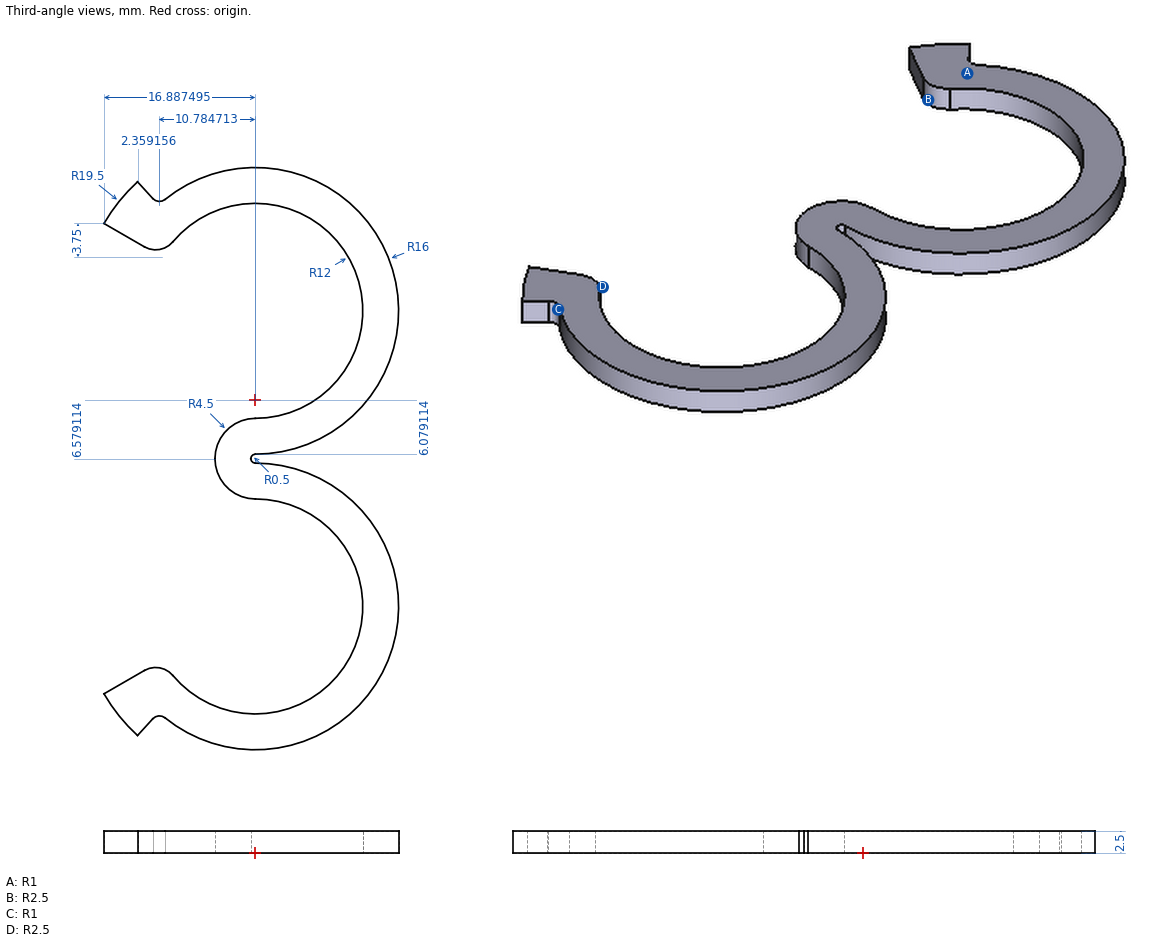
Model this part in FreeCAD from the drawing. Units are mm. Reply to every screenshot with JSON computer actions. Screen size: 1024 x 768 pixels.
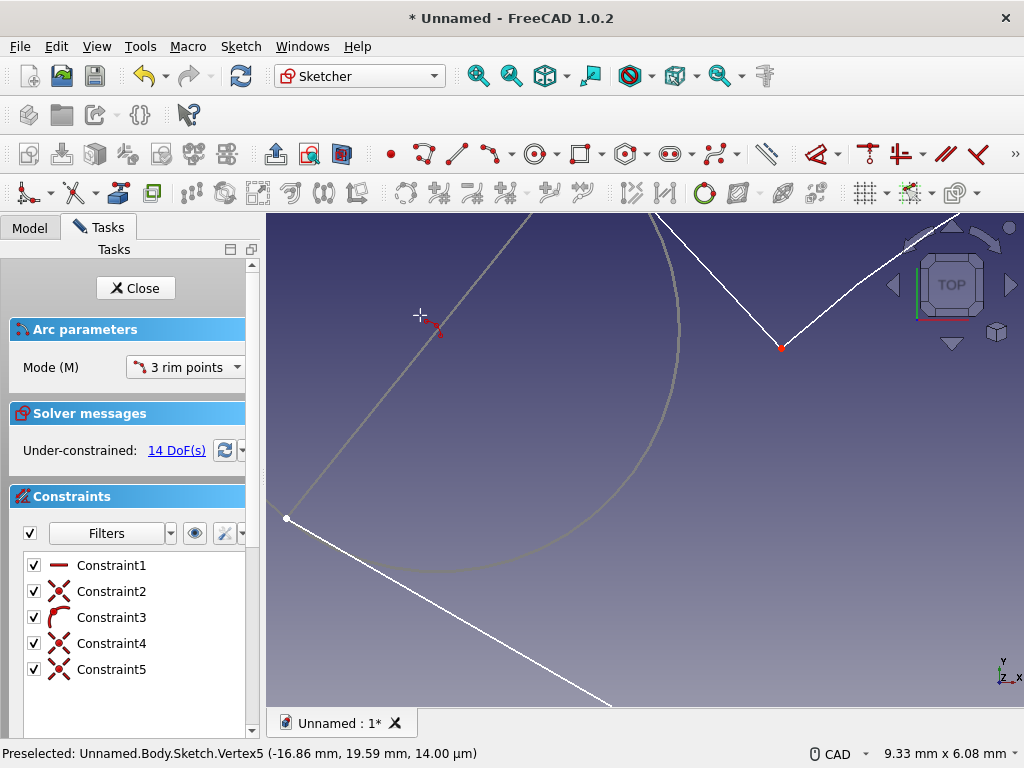
{"action": "left_click", "coordinate": [422, 311]}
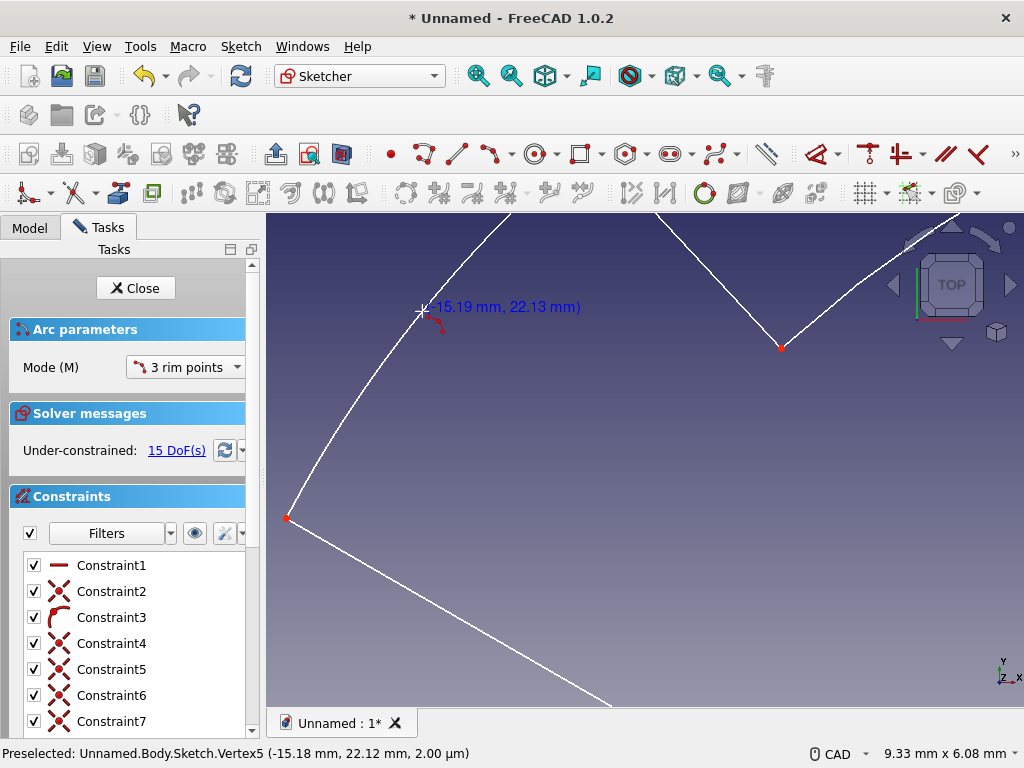
{"action": "scroll", "coordinate": [420, 315], "scroll_direction": "down", "scroll_amount": 10}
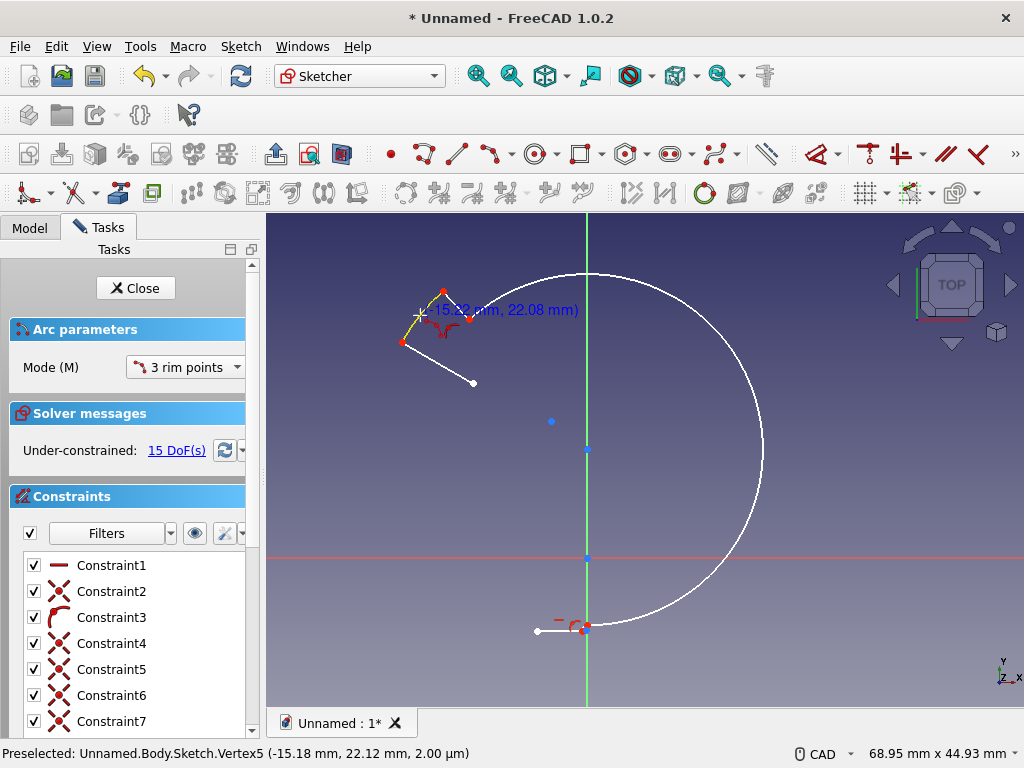
{"action": "left_click", "coordinate": [473, 384]}
{"action": "left_click", "coordinate": [587, 581]}
{"action": "left_click", "coordinate": [702, 383]}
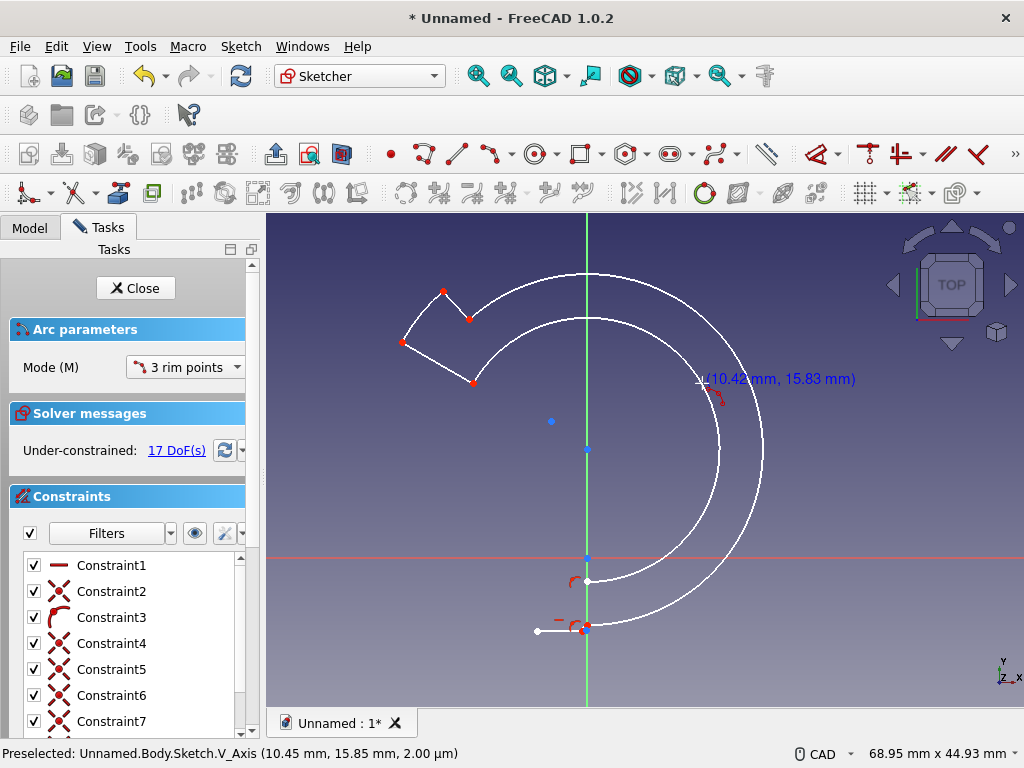
{"action": "left_click", "coordinate": [587, 582]}
{"action": "left_click", "coordinate": [538, 631]}
{"action": "left_click", "coordinate": [552, 595]}
{"action": "key", "text": "Escape"}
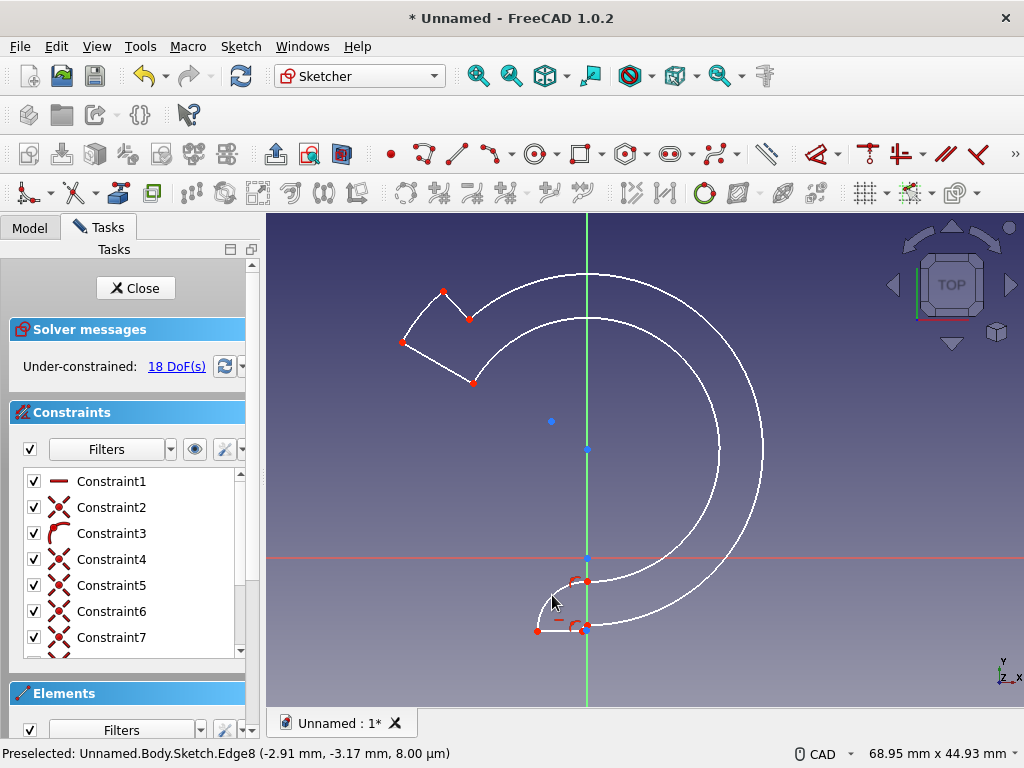
{"action": "scroll", "coordinate": [583, 627], "scroll_direction": "up", "scroll_amount": 6}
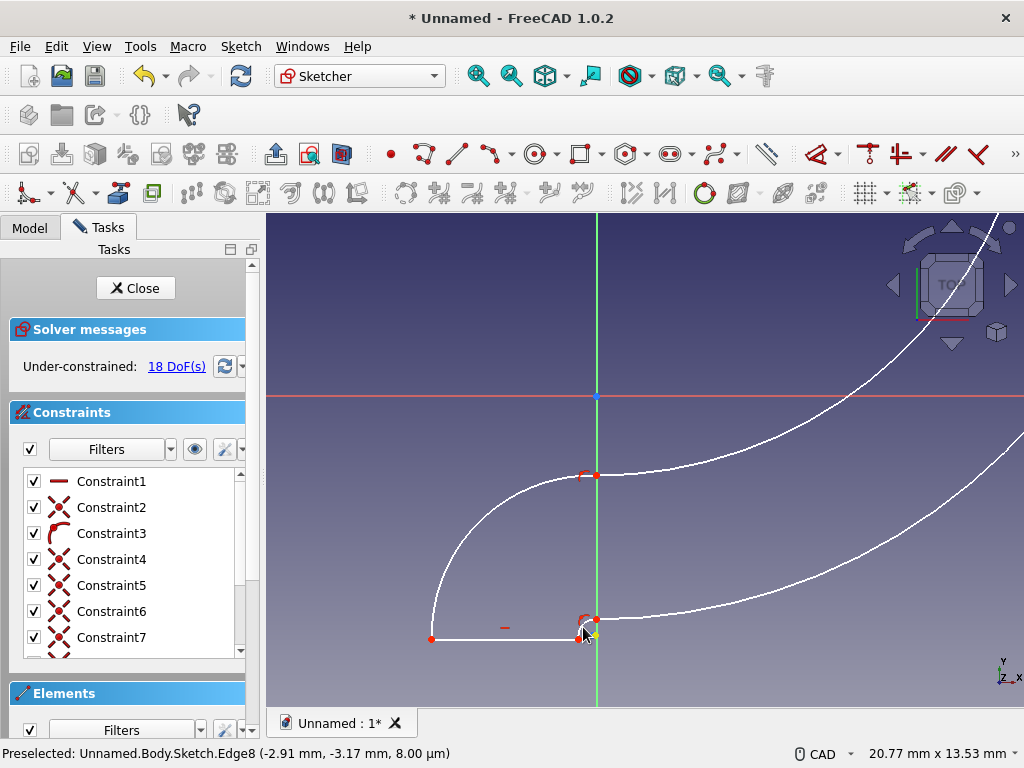
{"action": "left_click", "coordinate": [583, 625]}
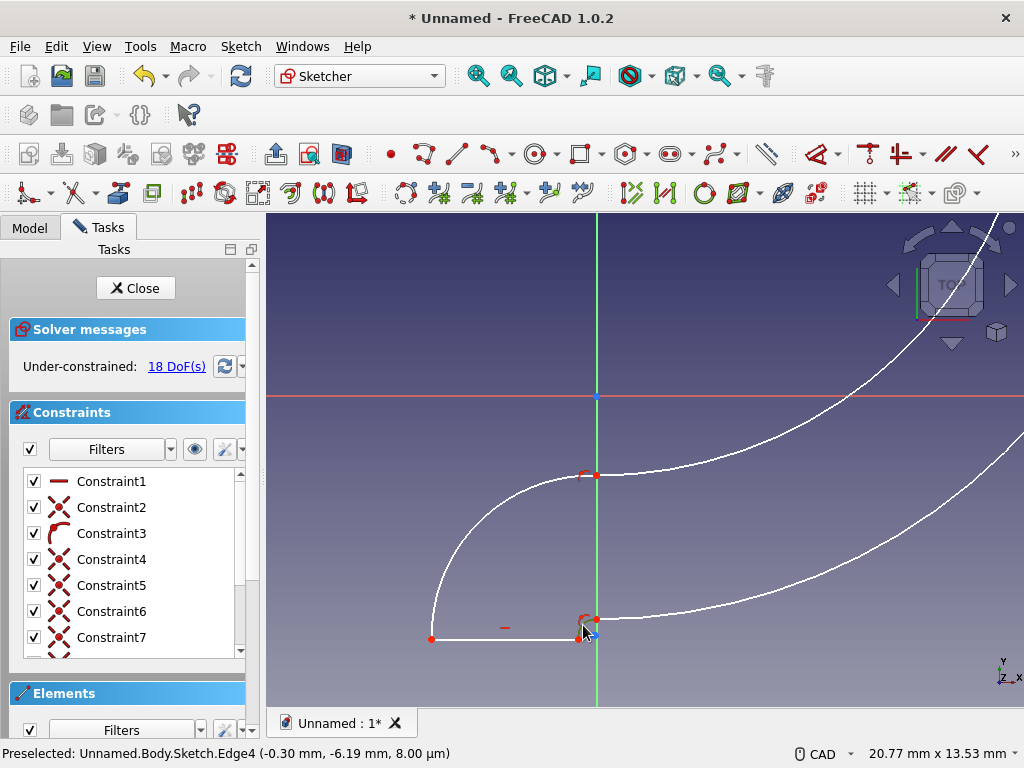
{"action": "scroll", "coordinate": [583, 627], "scroll_direction": "down", "scroll_amount": 6}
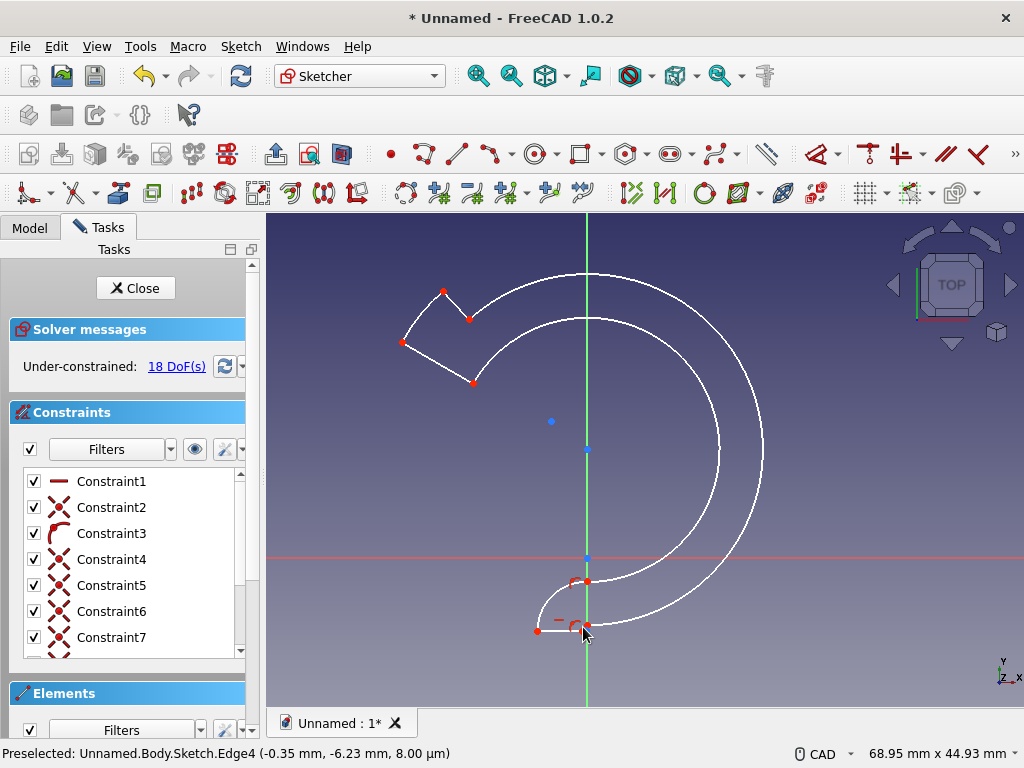
{"action": "left_click", "coordinate": [749, 519]}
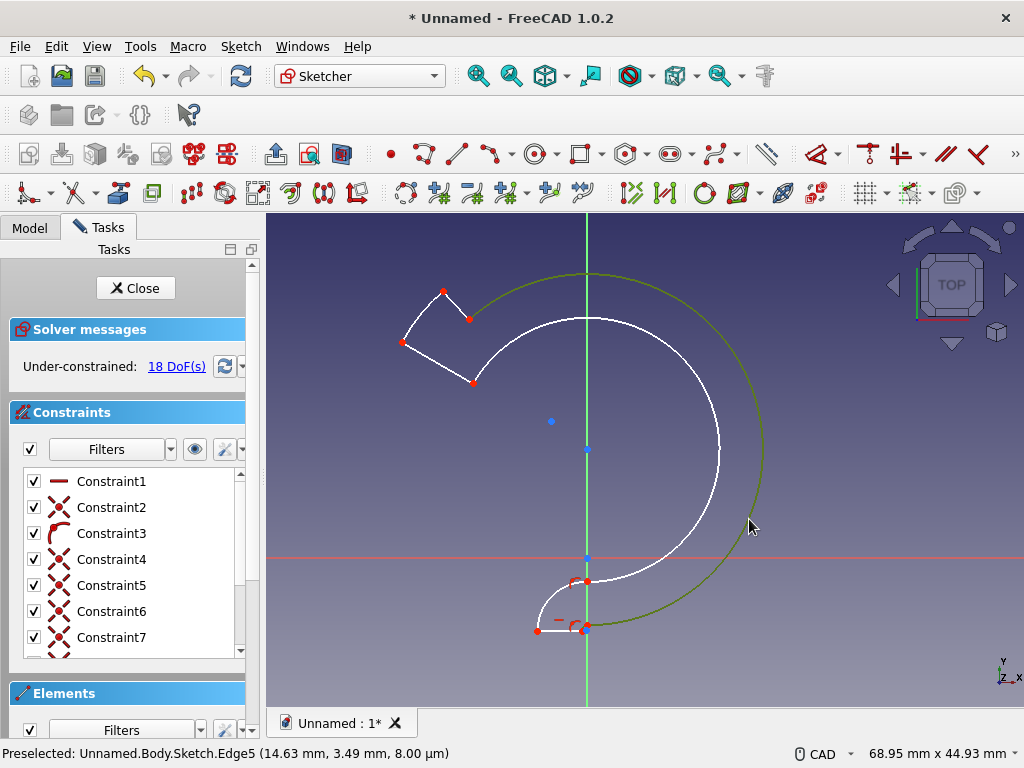
{"action": "key", "text": "t"}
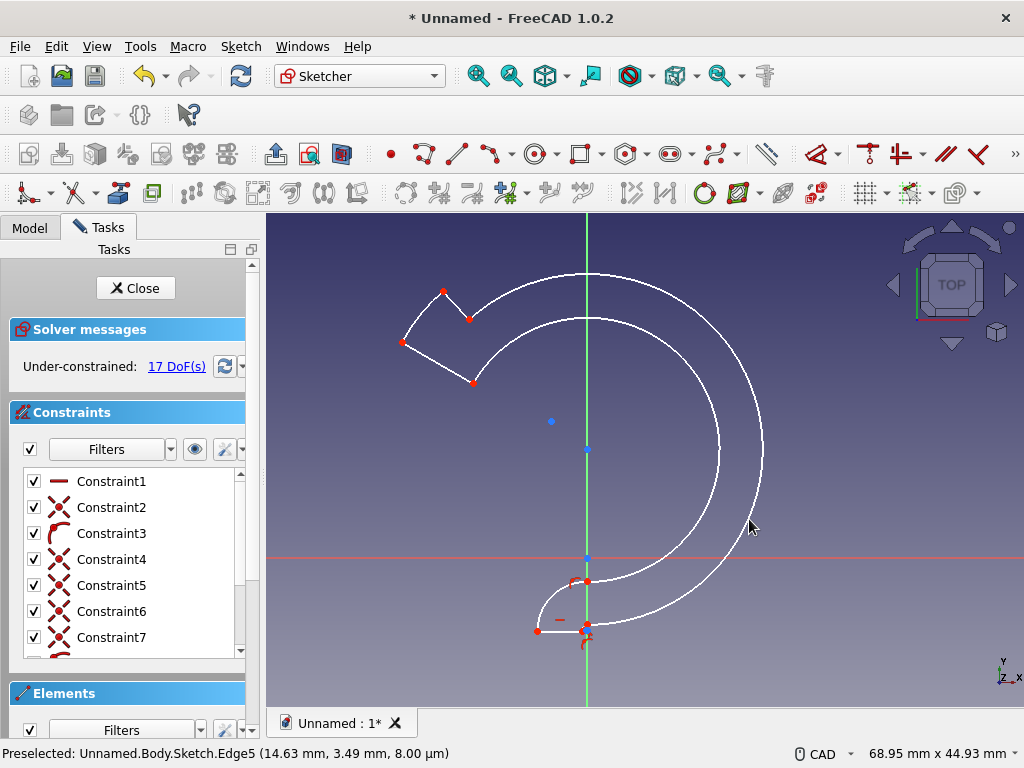
{"action": "left_click", "coordinate": [713, 491]}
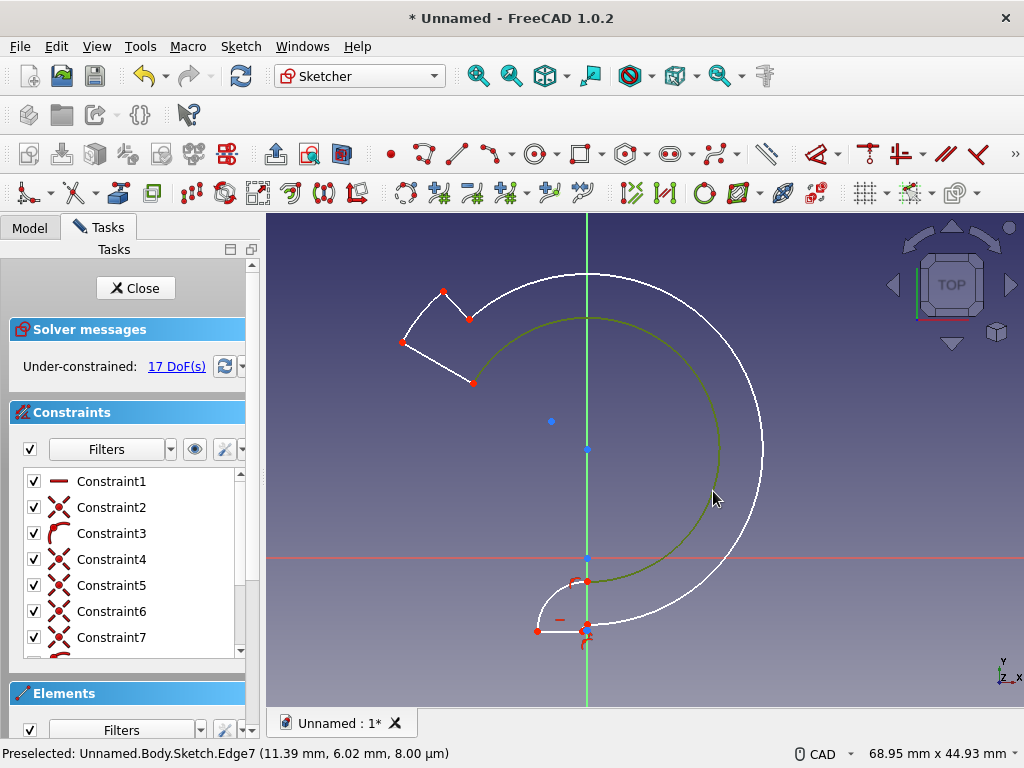
{"action": "left_click", "coordinate": [565, 587]}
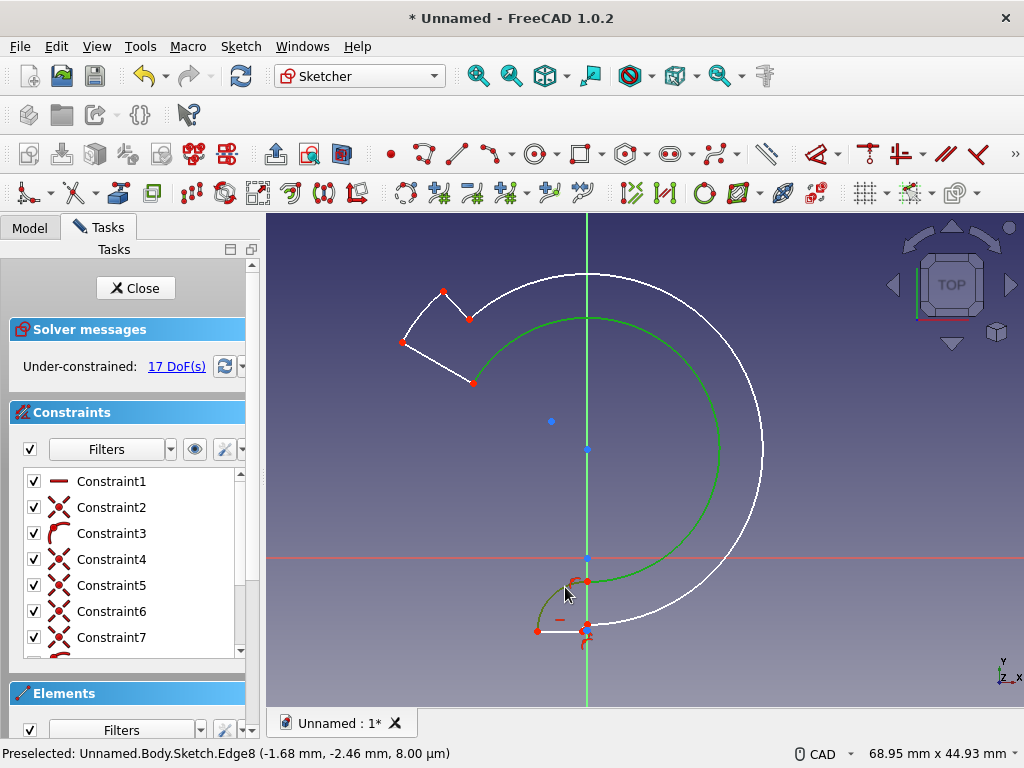
{"action": "key", "text": "t"}